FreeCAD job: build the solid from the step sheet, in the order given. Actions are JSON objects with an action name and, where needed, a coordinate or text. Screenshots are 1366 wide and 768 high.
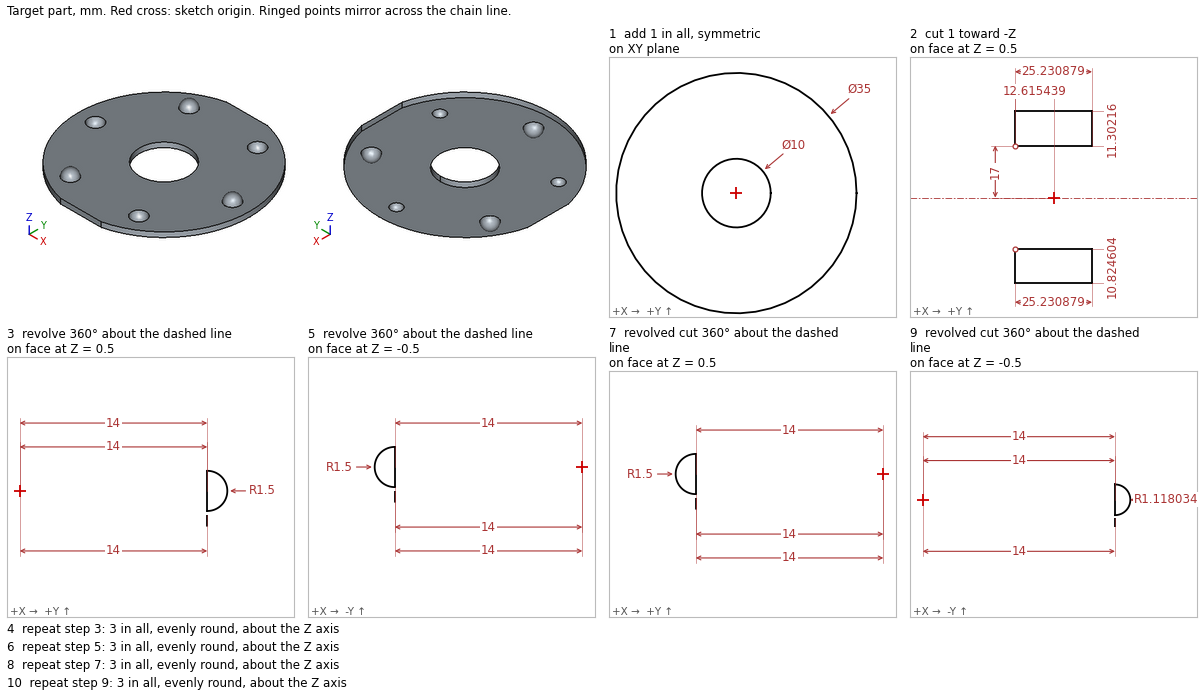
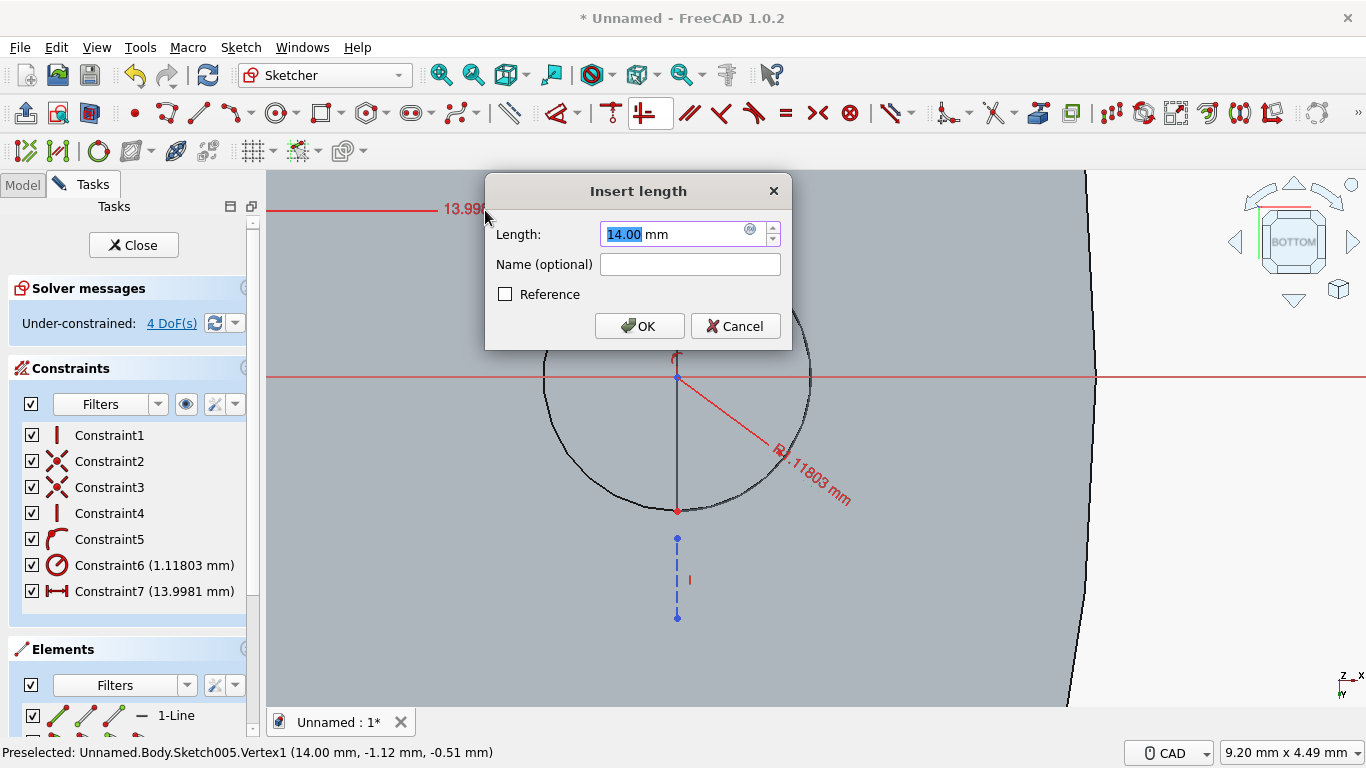
{"action": "type", "text": "14"}
{"action": "key", "text": "Return"}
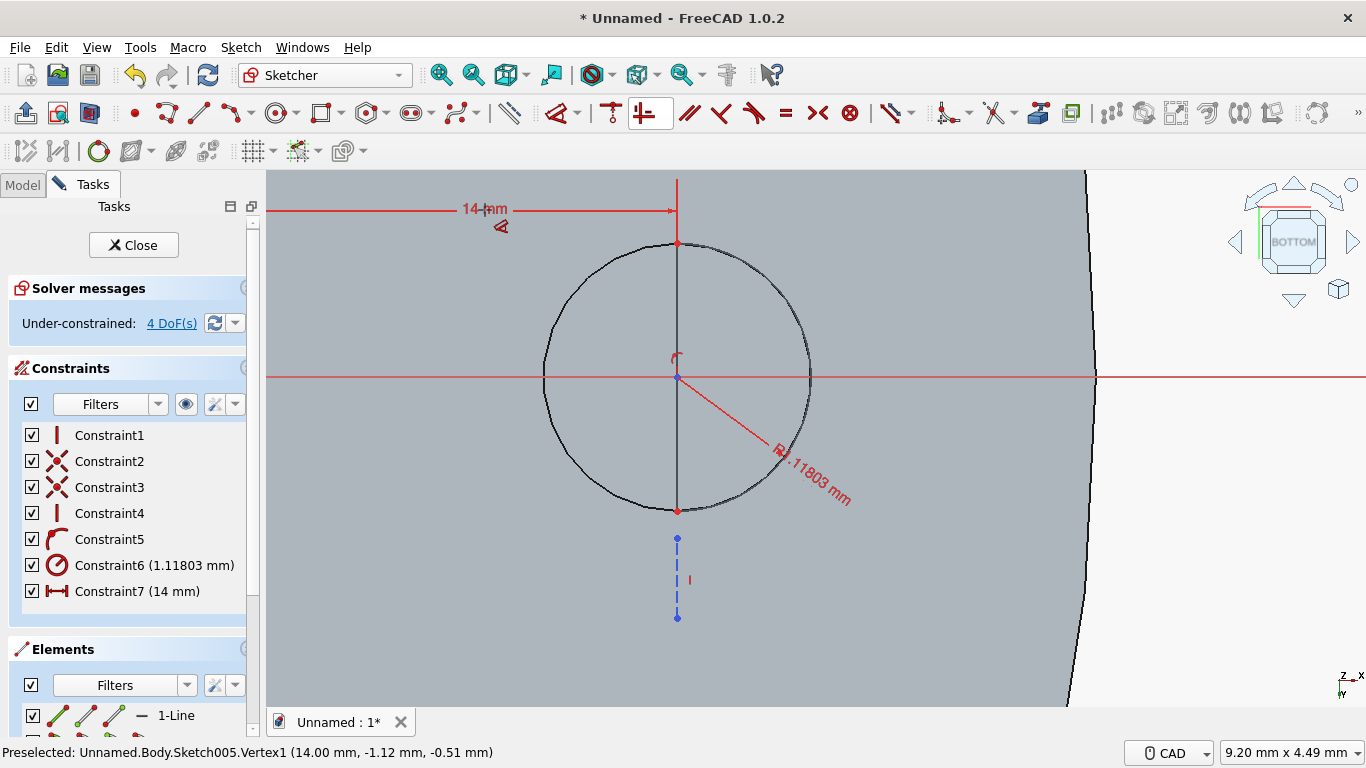
{"action": "left_click", "coordinate": [677, 539]}
{"action": "left_click", "coordinate": [486, 573]}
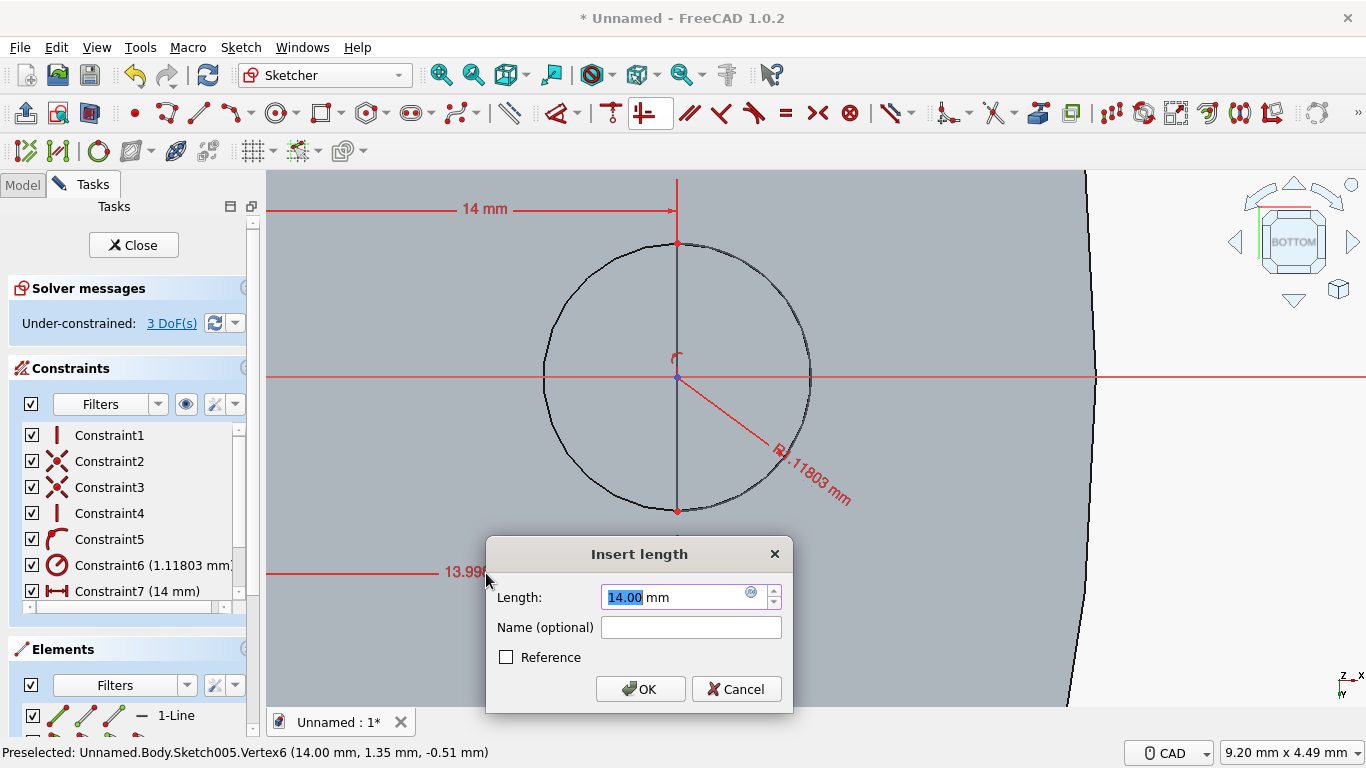
{"action": "type", "text": "14"}
{"action": "key", "text": "Return"}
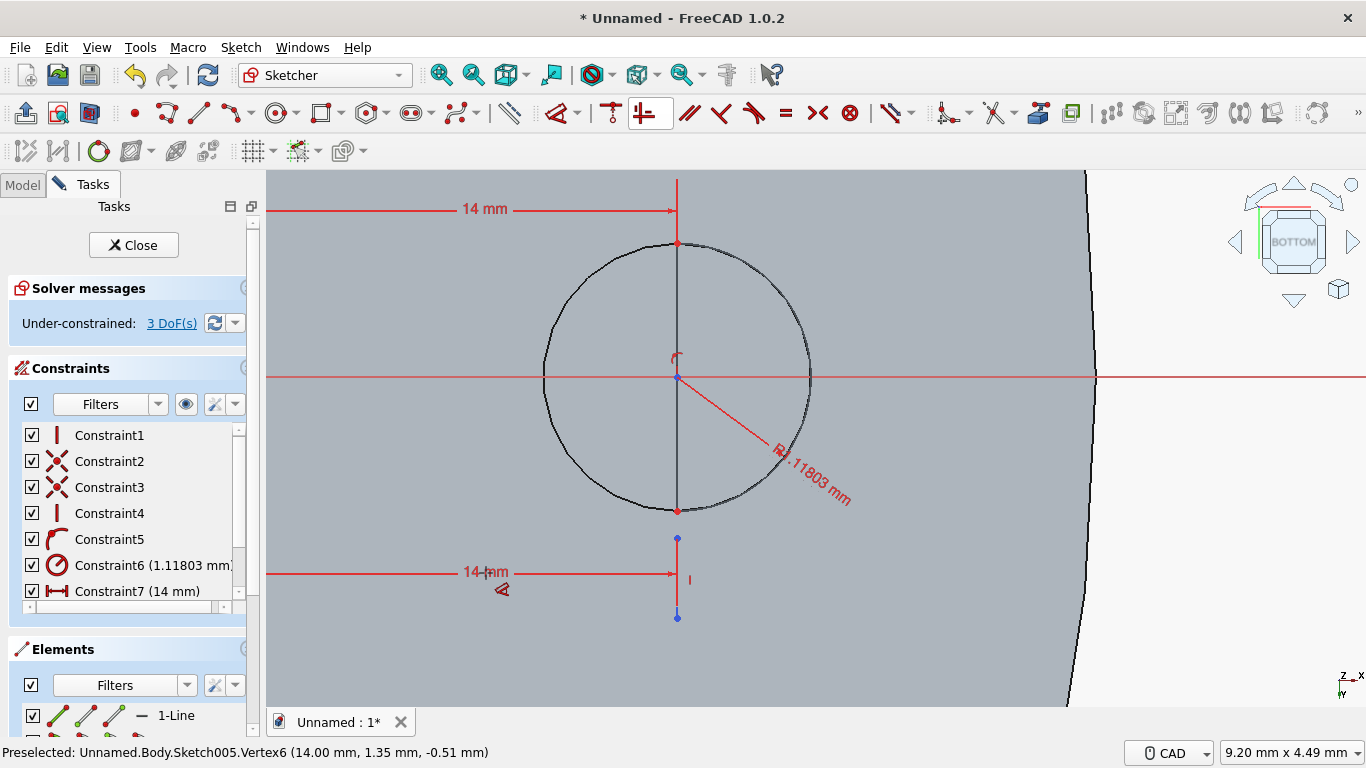
{"action": "left_click", "coordinate": [677, 377]}
{"action": "left_click", "coordinate": [486, 343]}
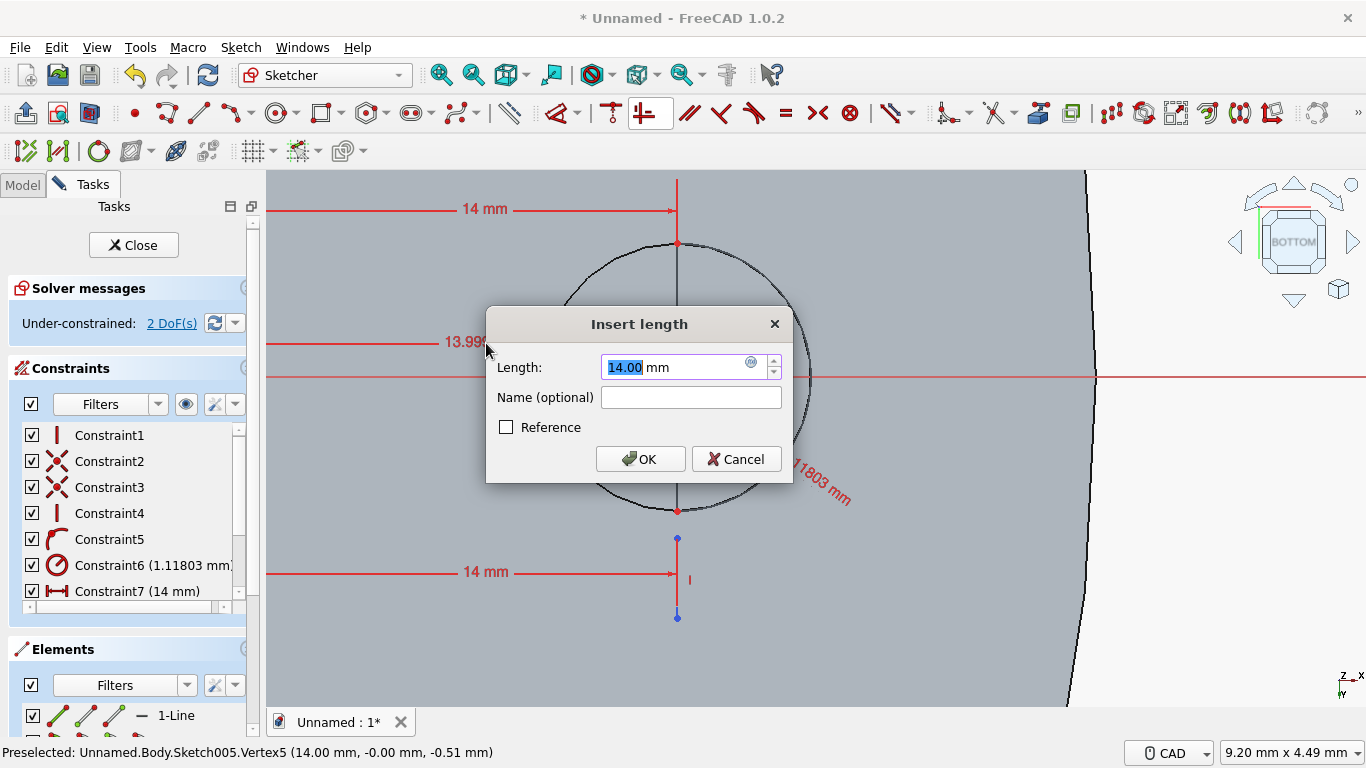
{"action": "type", "text": "14"}
{"action": "key", "text": "Return"}
{"action": "key", "text": "Escape"}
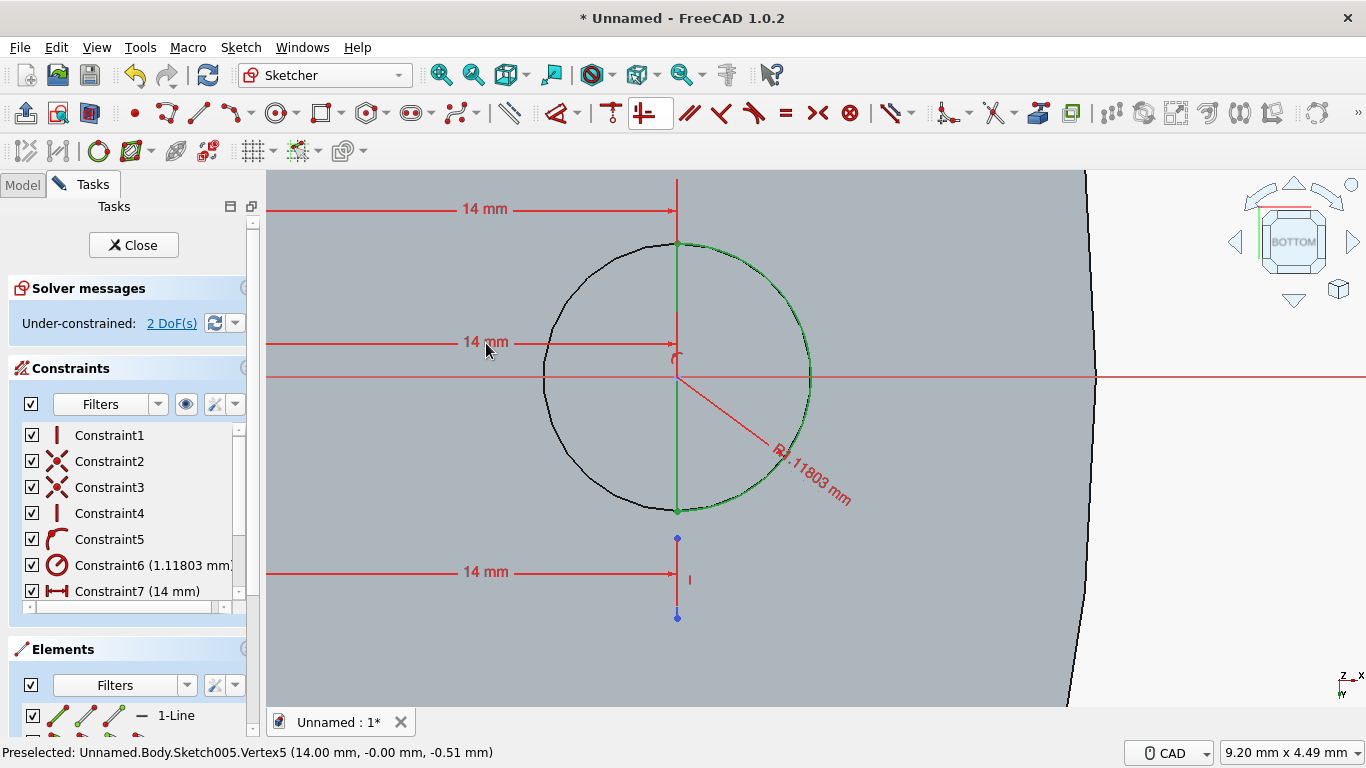
{"action": "left_click", "coordinate": [134, 245]}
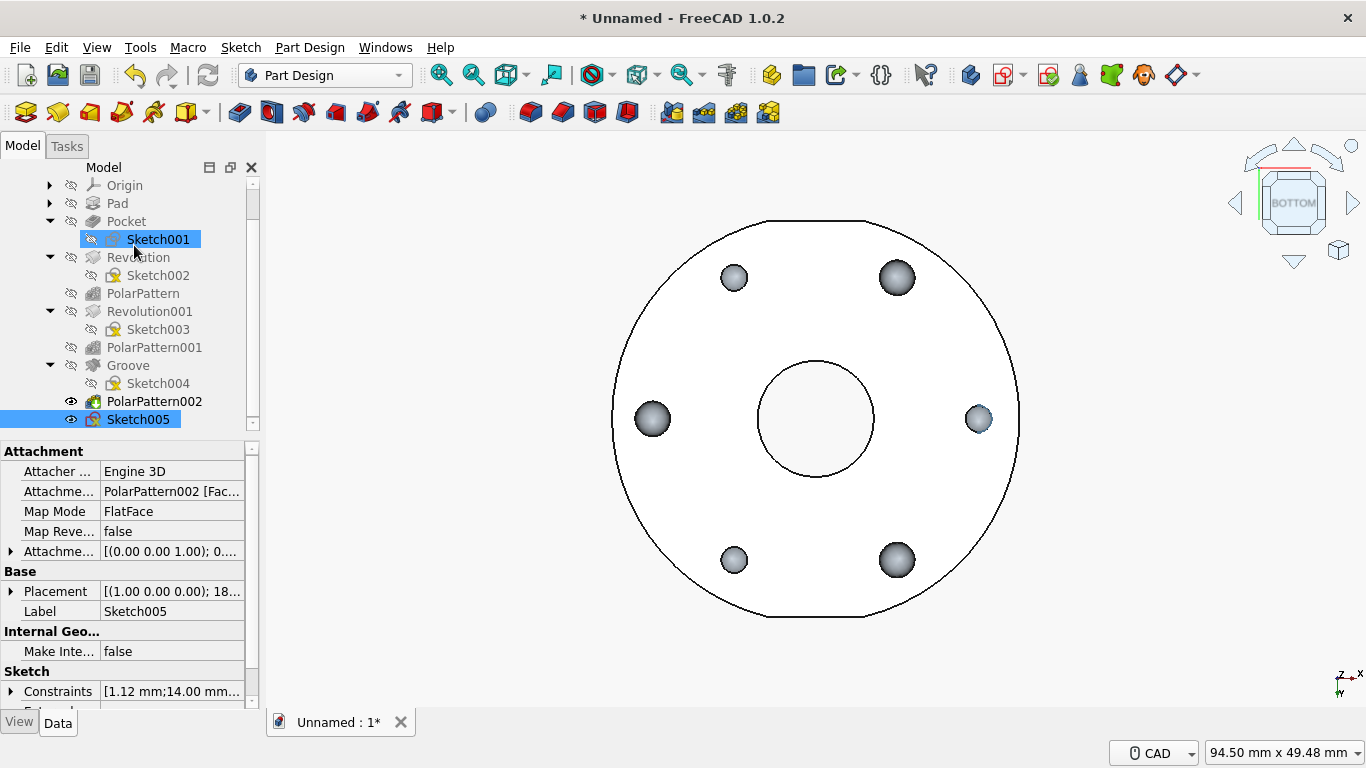
{"action": "left_click", "coordinate": [304, 112]}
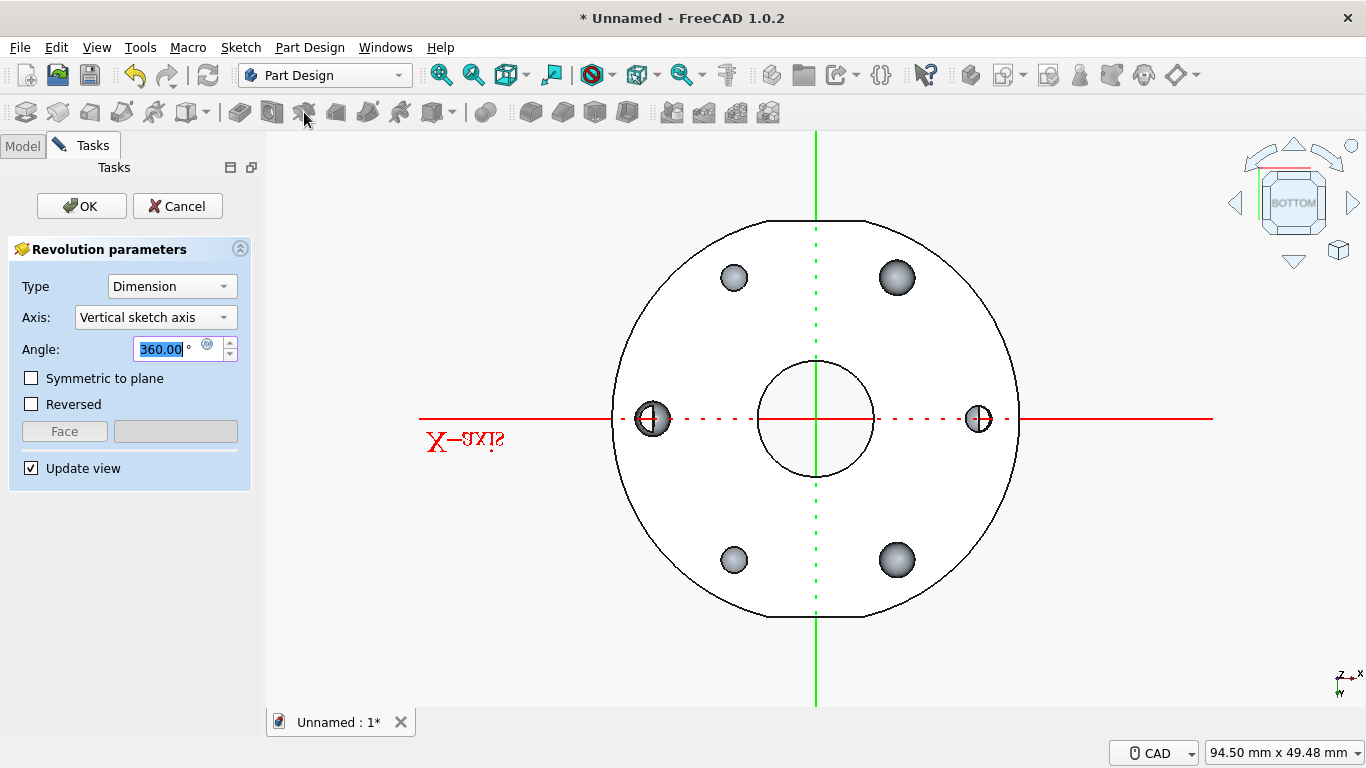
{"action": "left_click", "coordinate": [156, 318]}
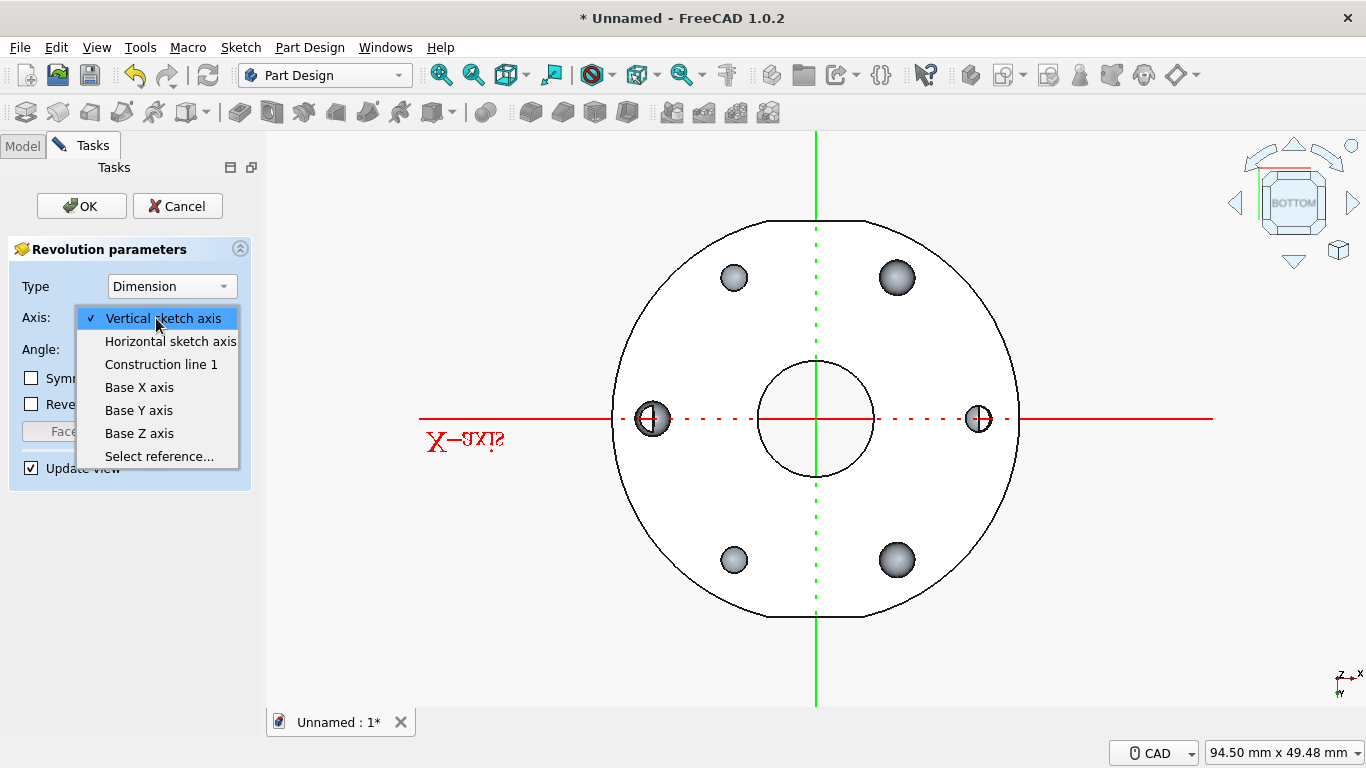
{"action": "left_click", "coordinate": [156, 364]}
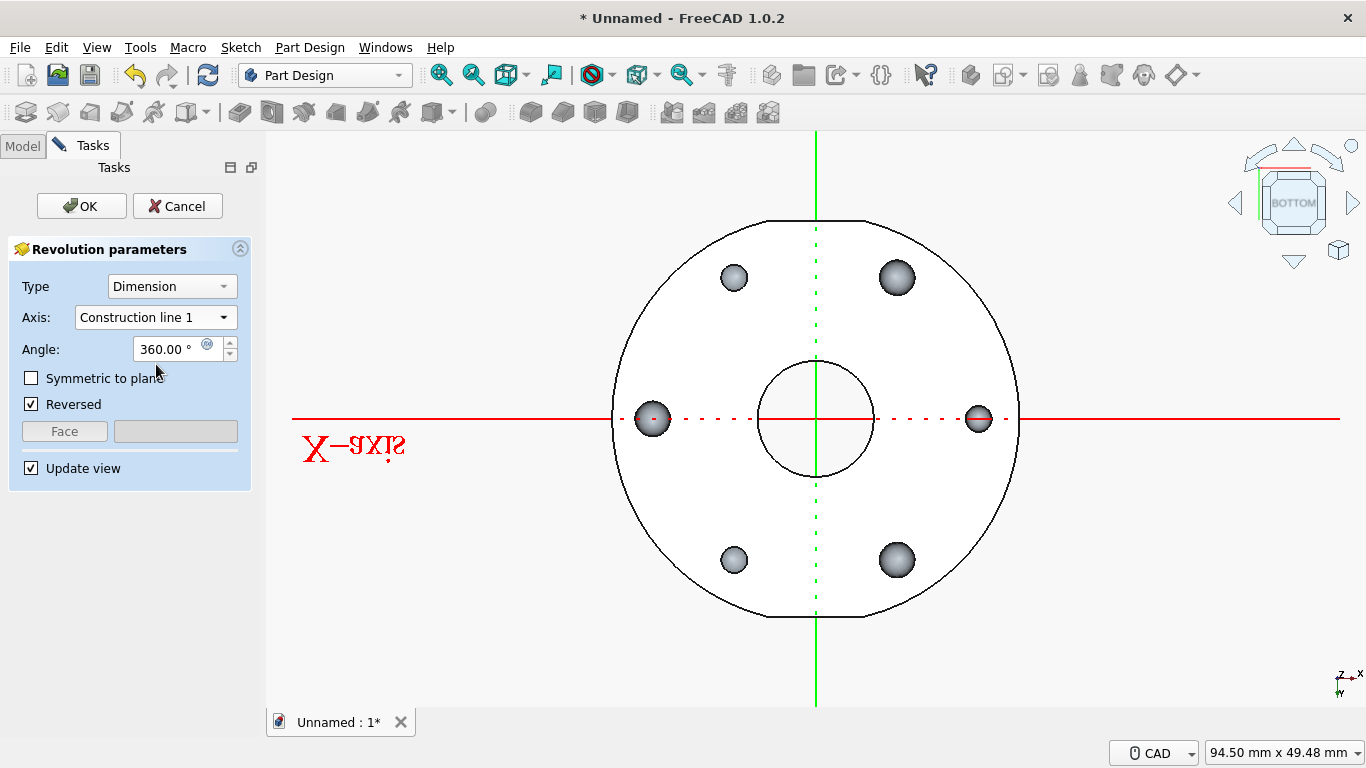
{"action": "left_click", "coordinate": [82, 206]}